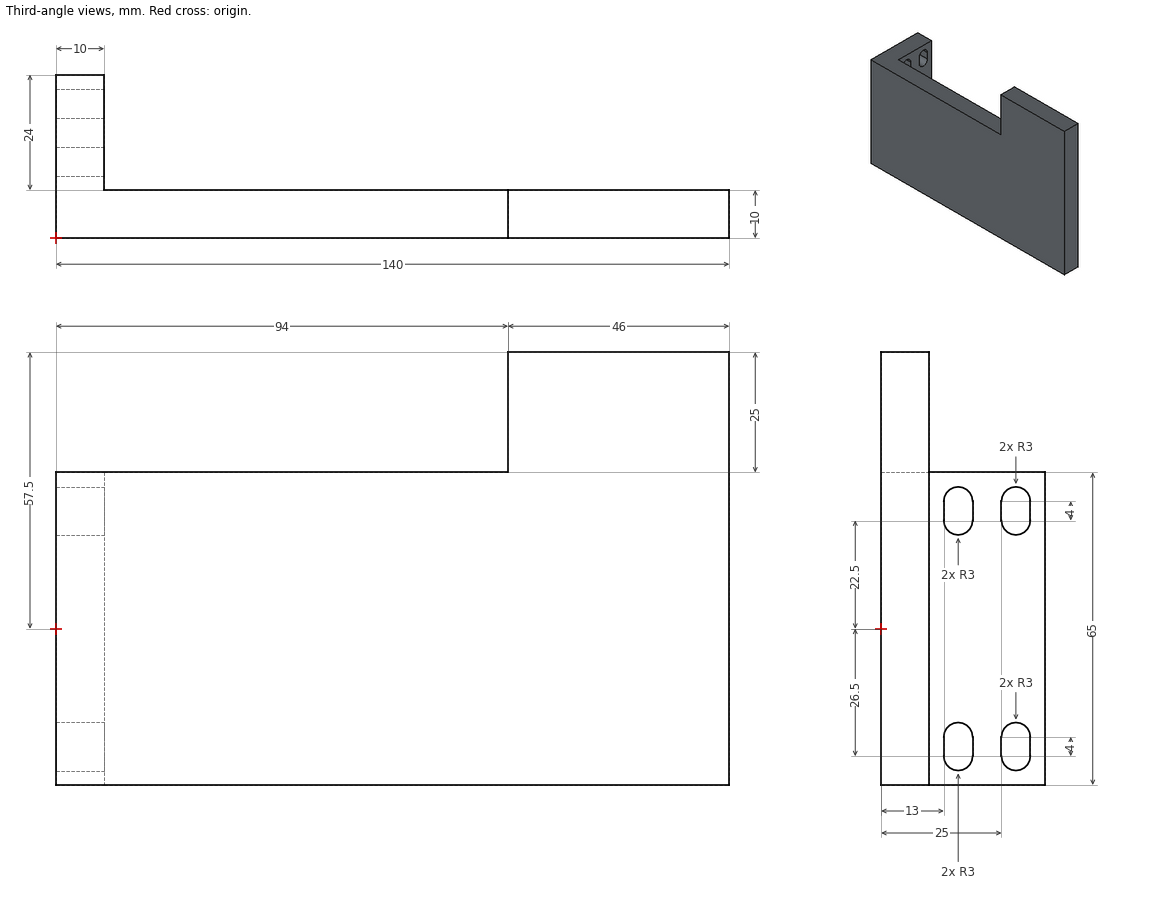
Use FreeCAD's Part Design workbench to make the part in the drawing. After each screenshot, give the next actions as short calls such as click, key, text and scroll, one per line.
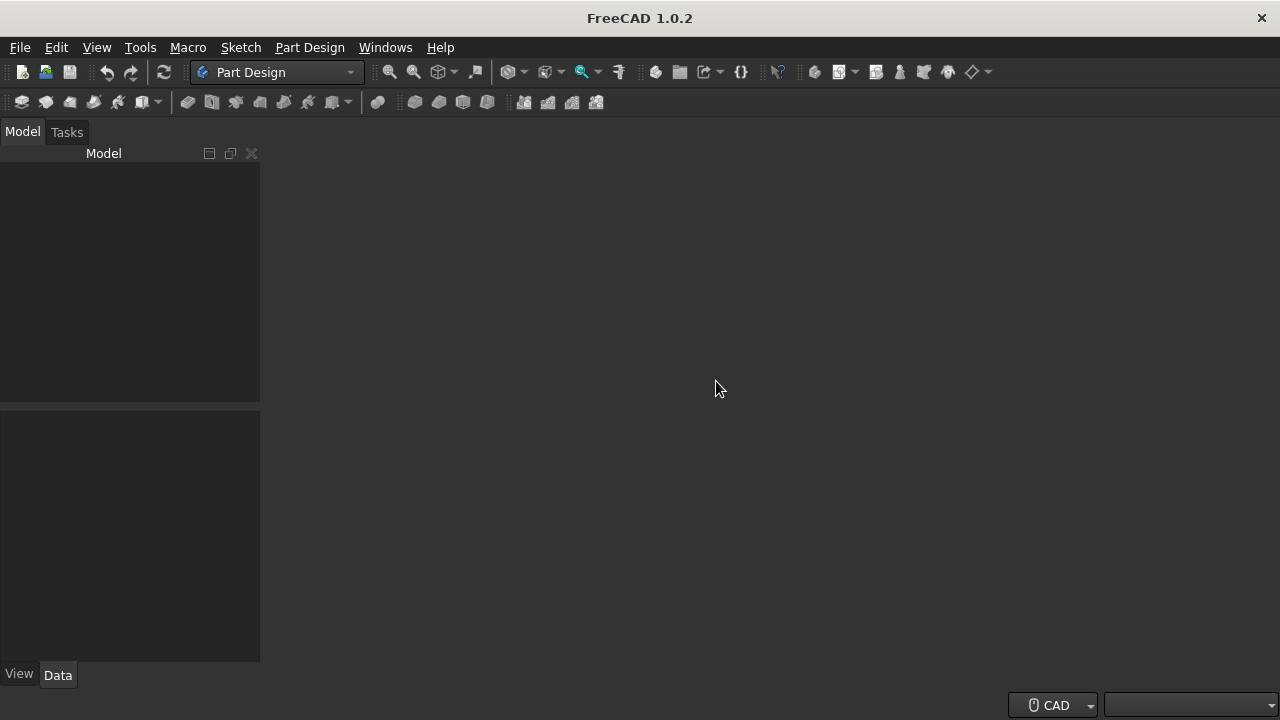
click(22, 72)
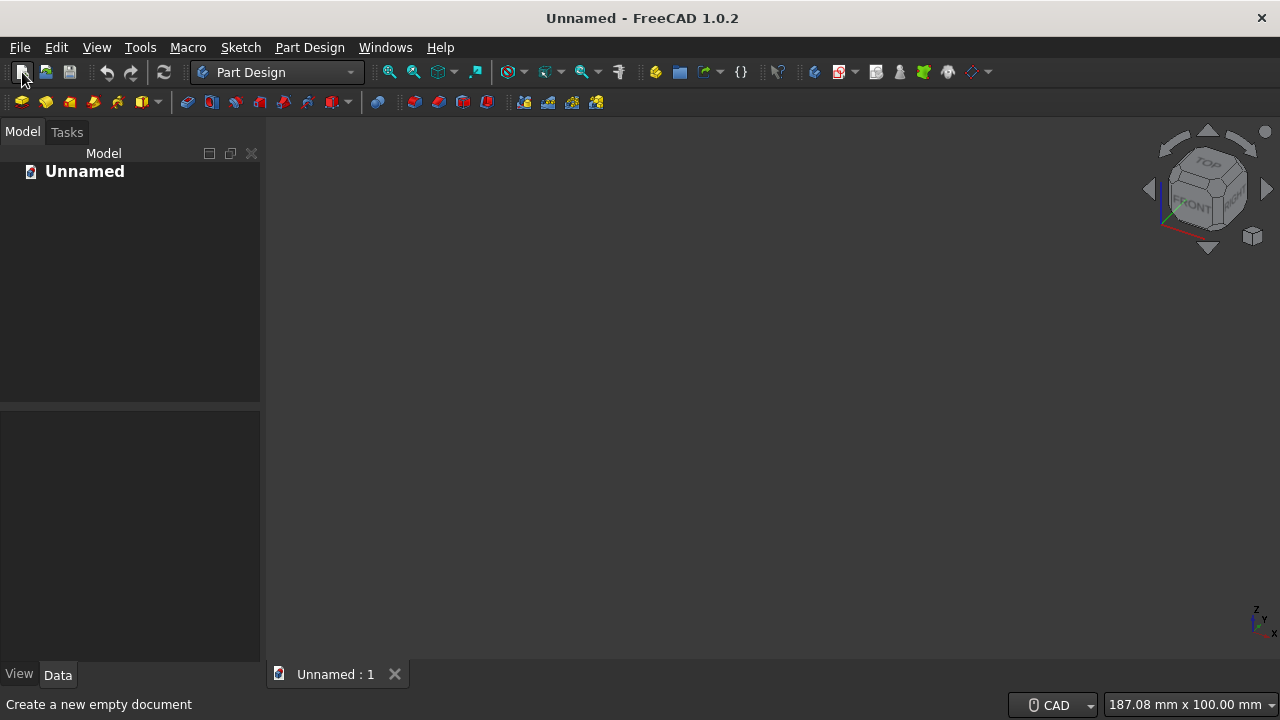
click(840, 72)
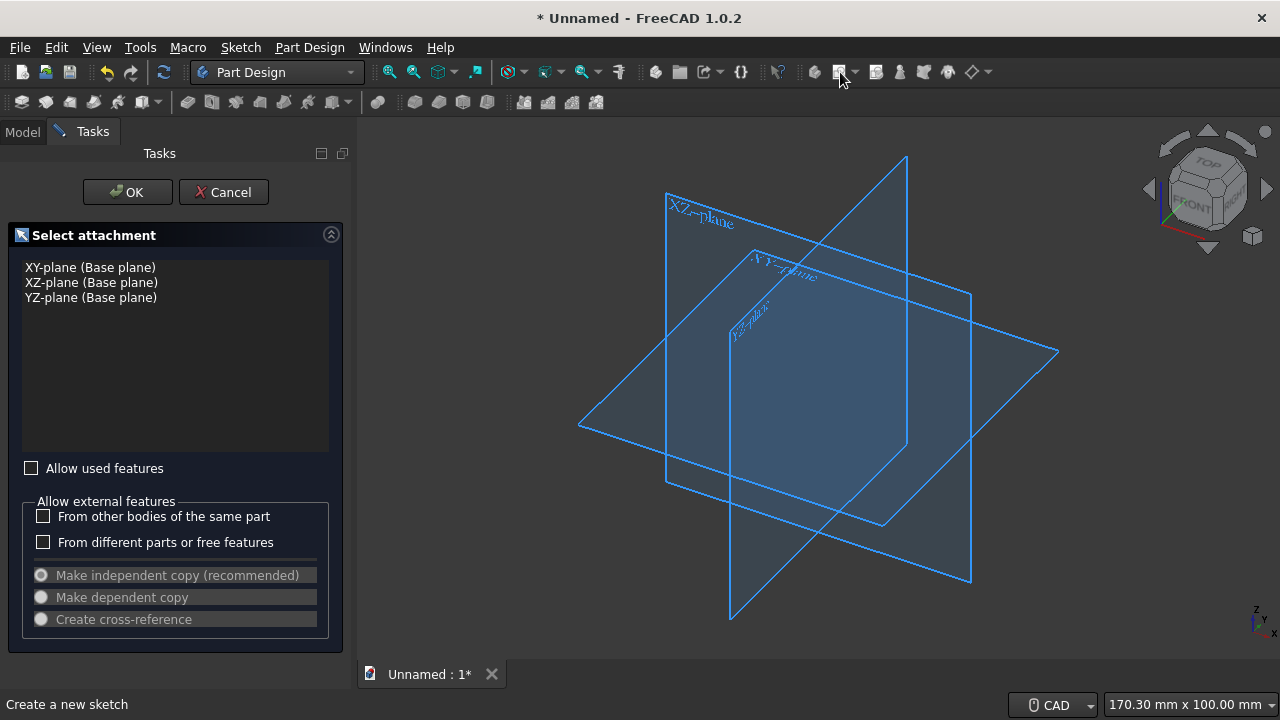
click(82, 268)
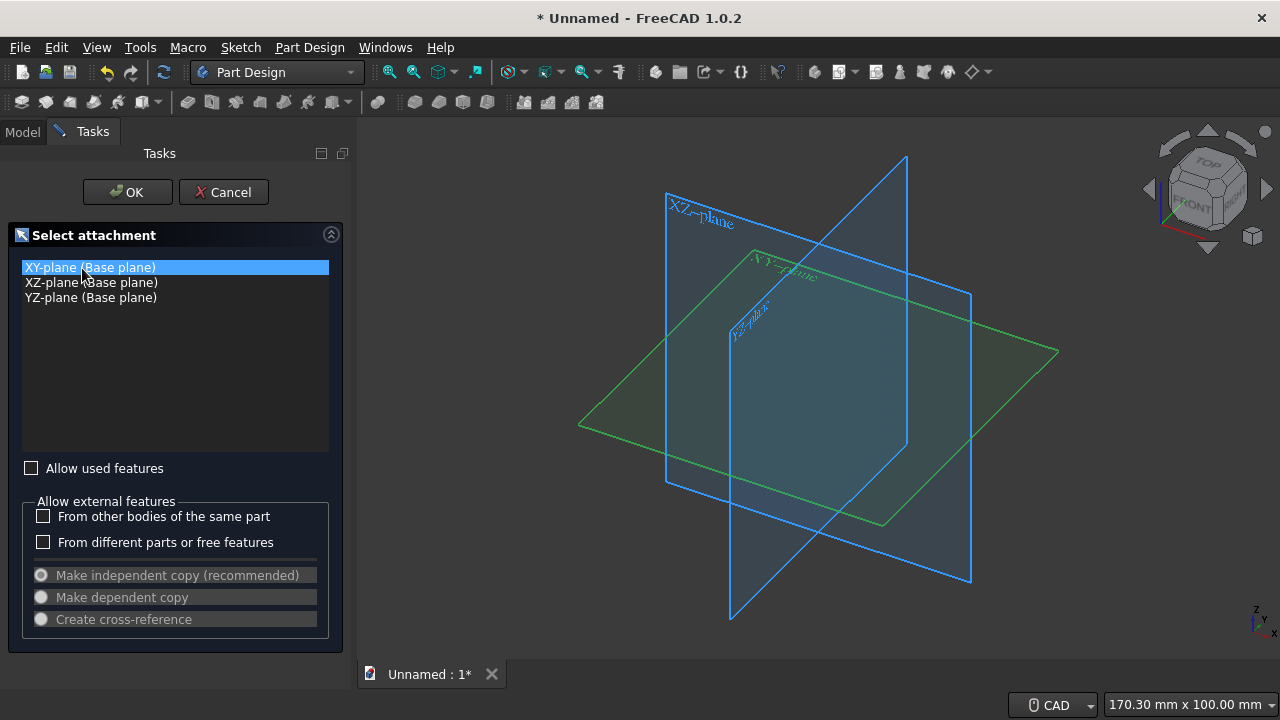
click(128, 192)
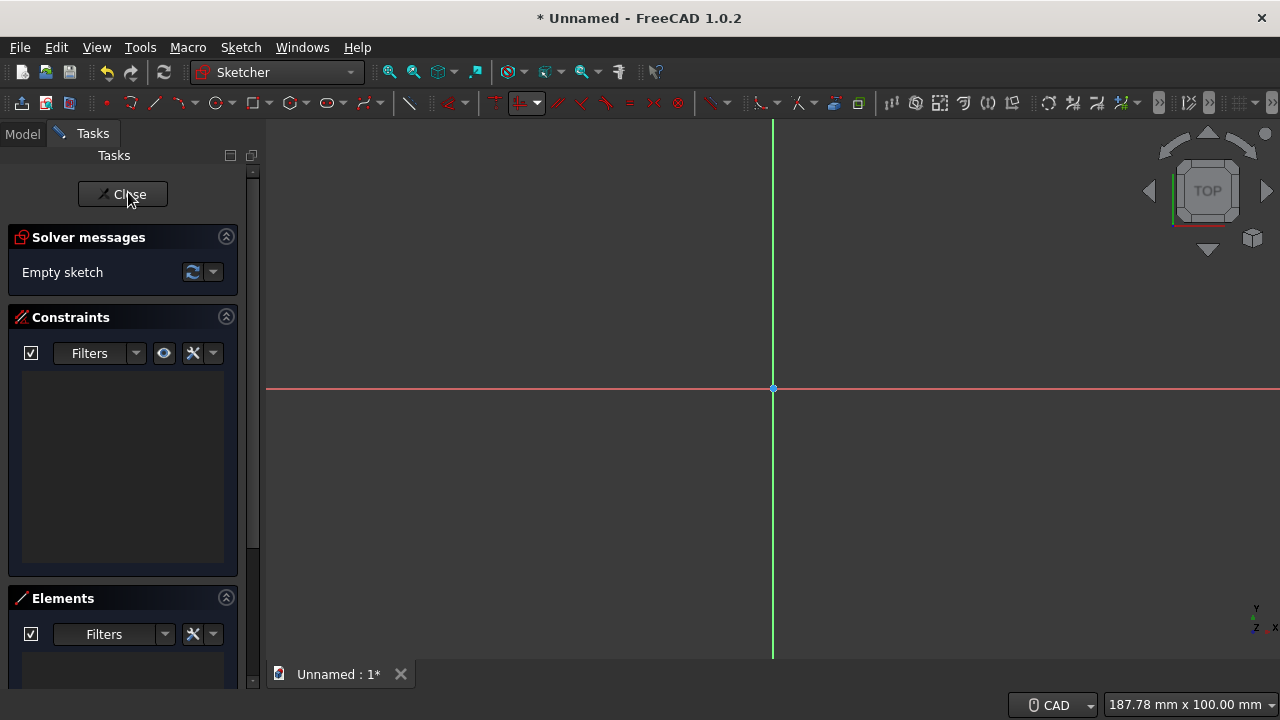
scroll(294, 501, down, 3)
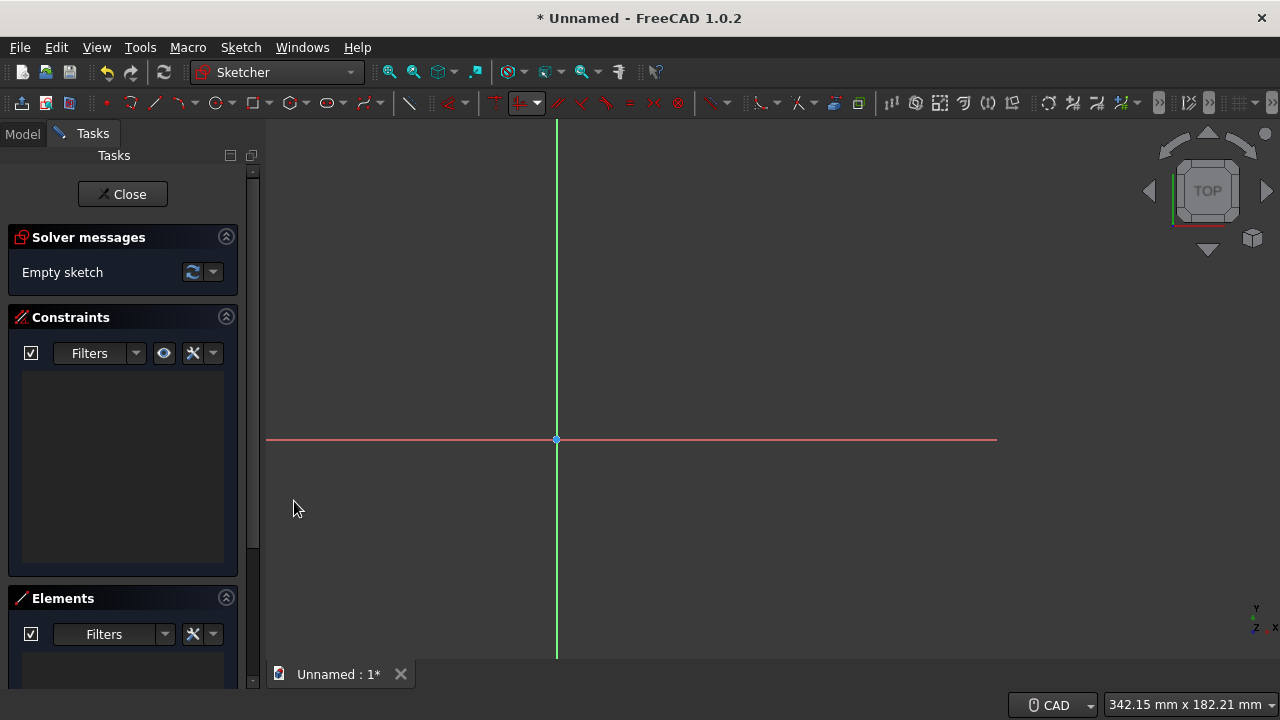
scroll(886, 390, up, 2)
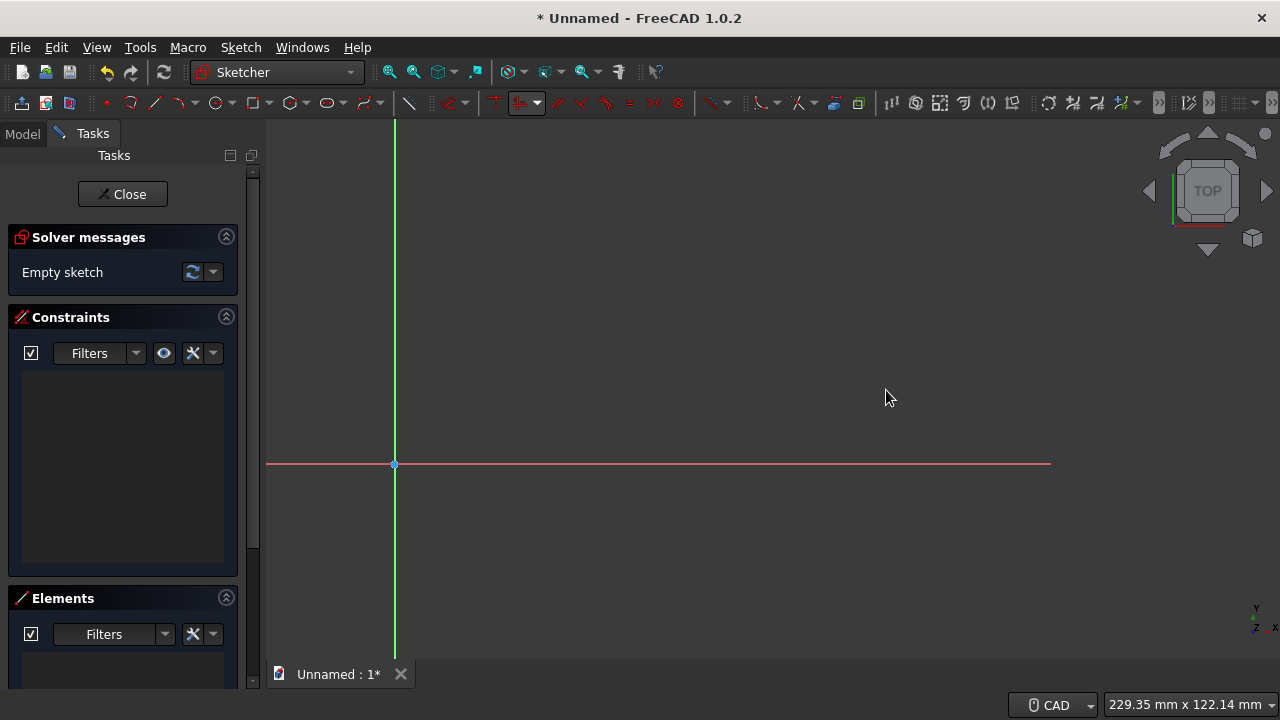
key(g)
key(m)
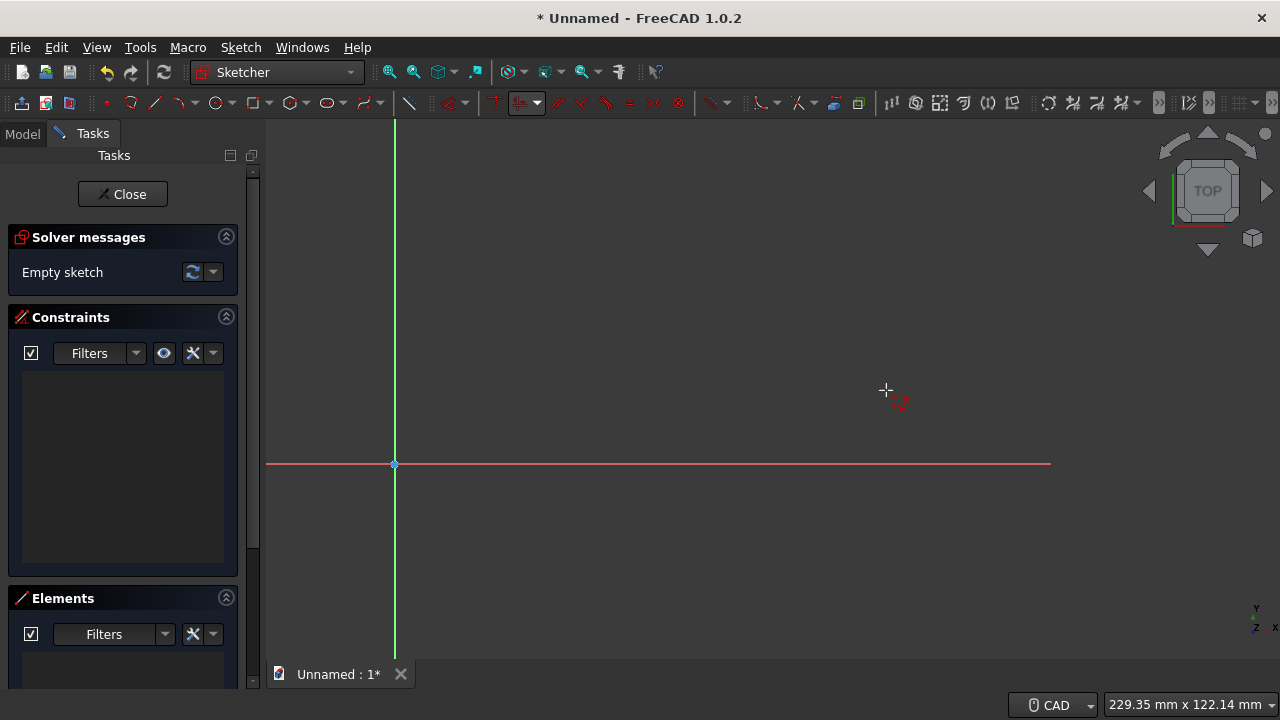
click(395, 464)
click(1014, 455)
click(1014, 420)
click(439, 420)
click(439, 314)
click(404, 314)
click(395, 464)
key(Escape)
key(Escape)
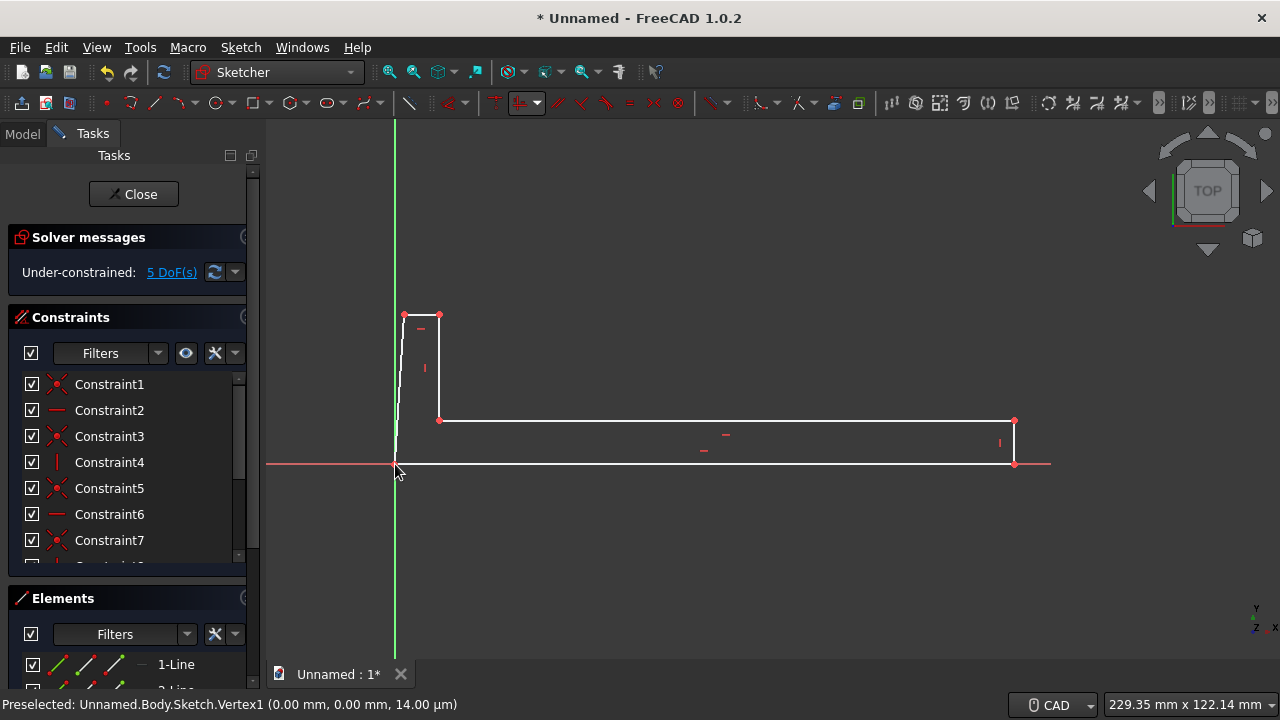
click(398, 419)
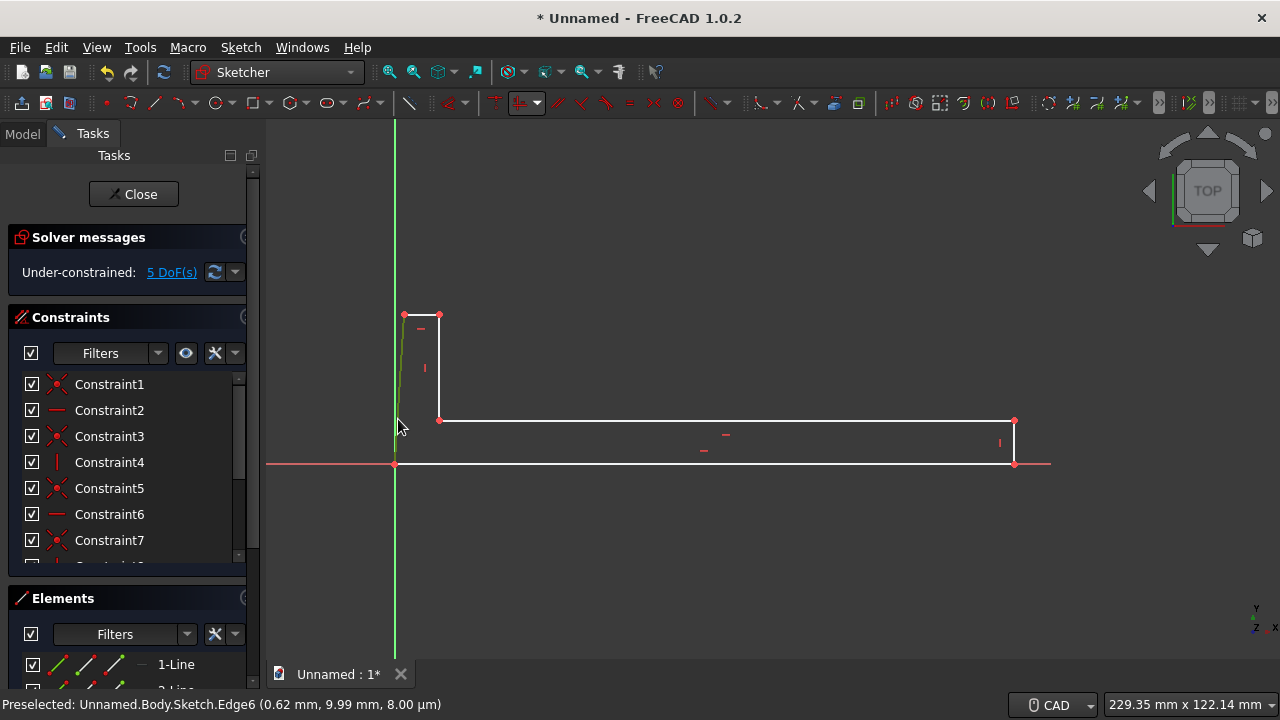
click(540, 104)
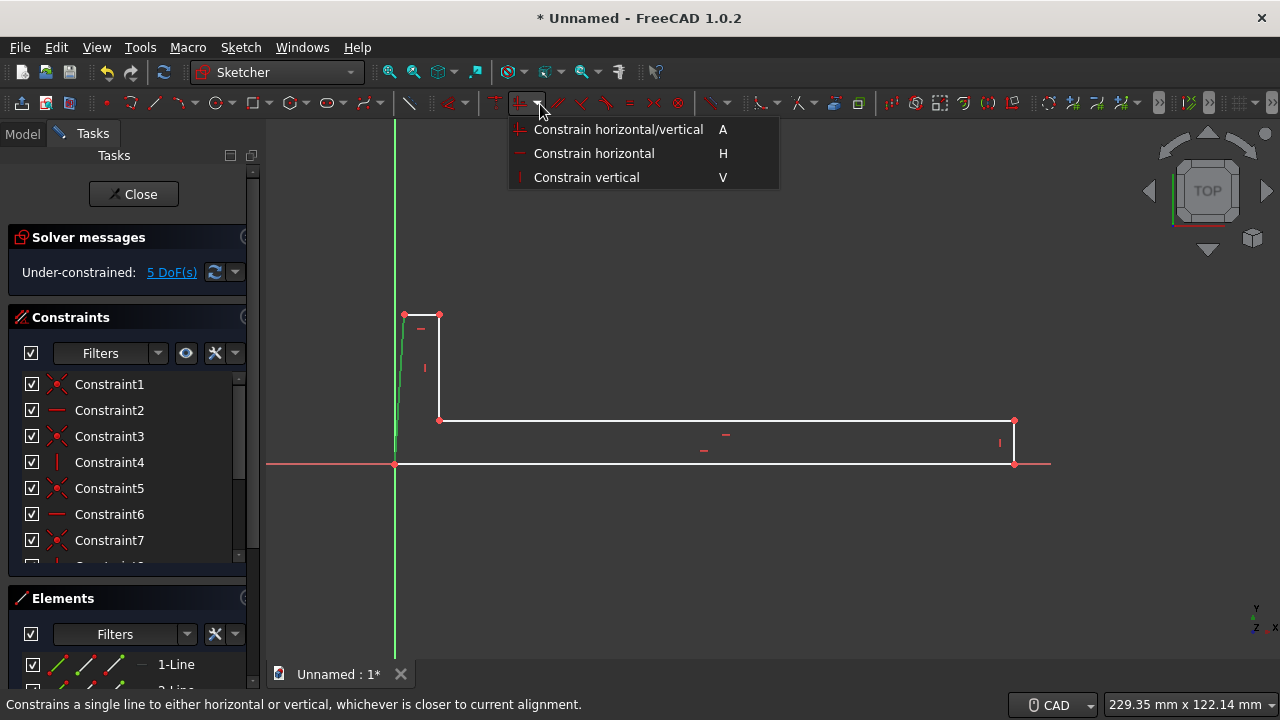
click(644, 177)